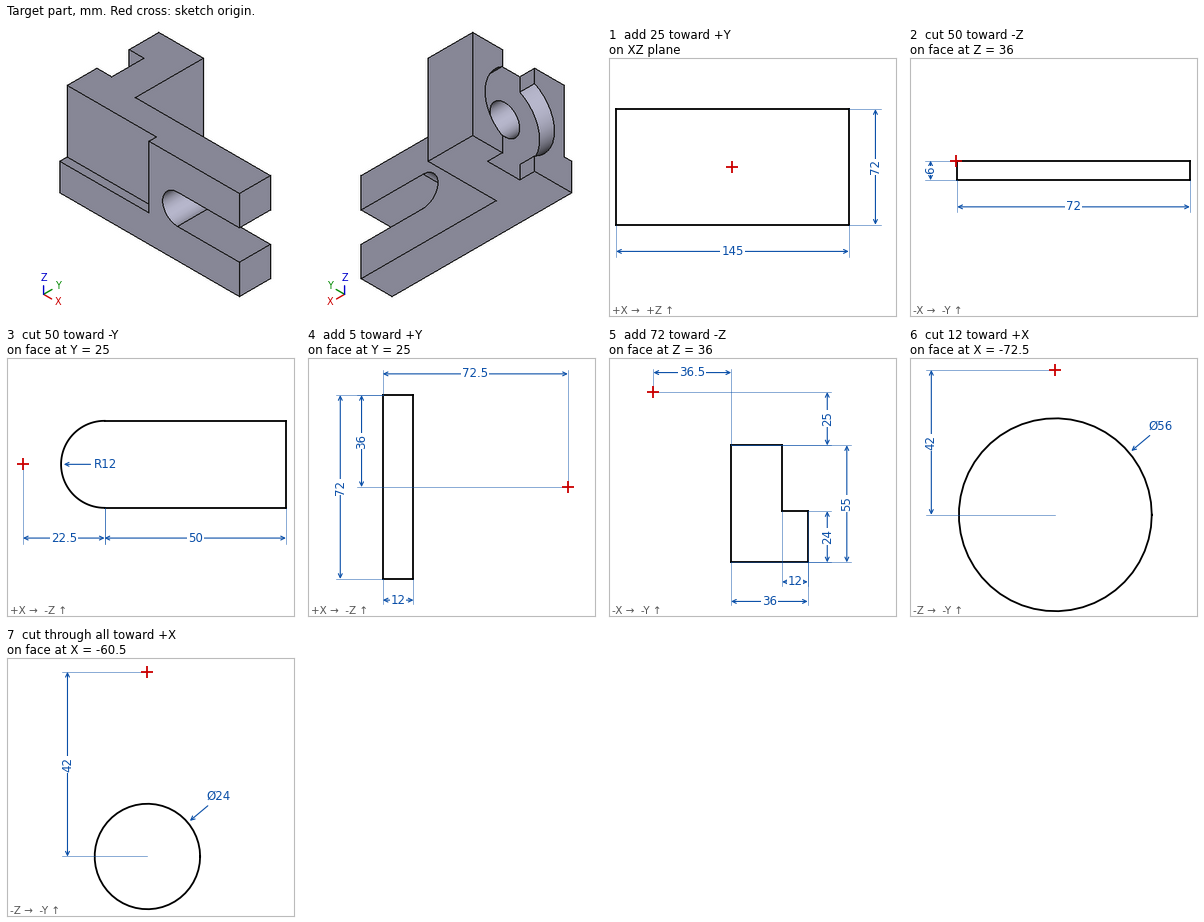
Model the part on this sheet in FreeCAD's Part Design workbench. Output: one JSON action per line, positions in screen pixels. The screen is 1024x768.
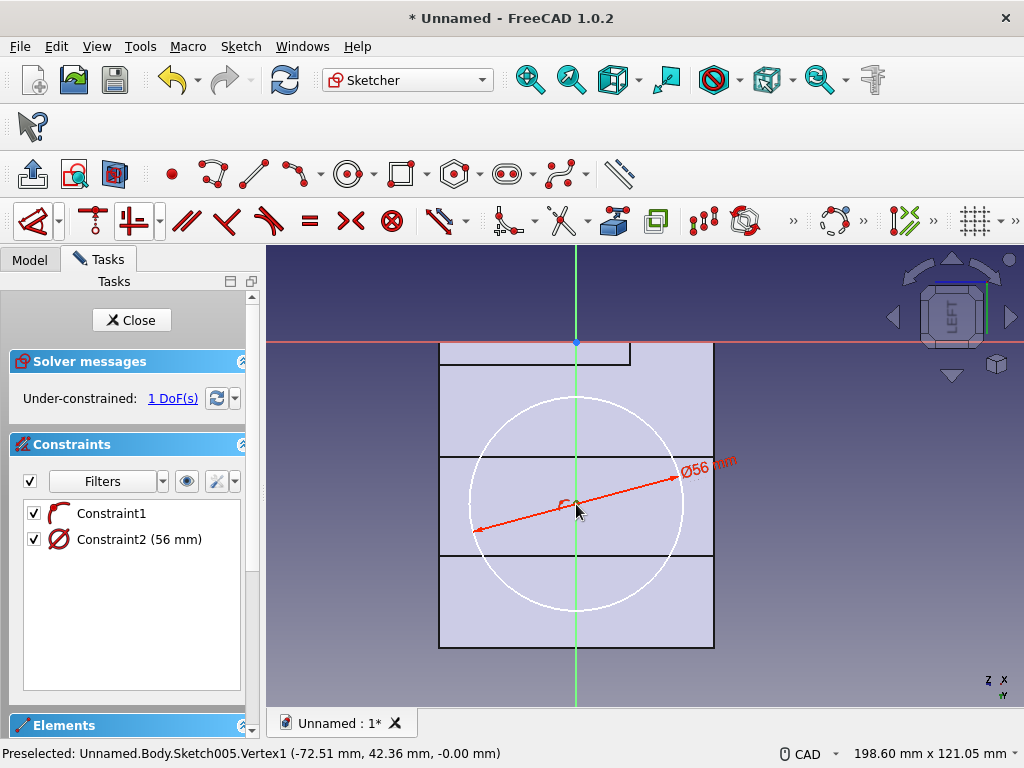
{"action": "key", "text": "i"}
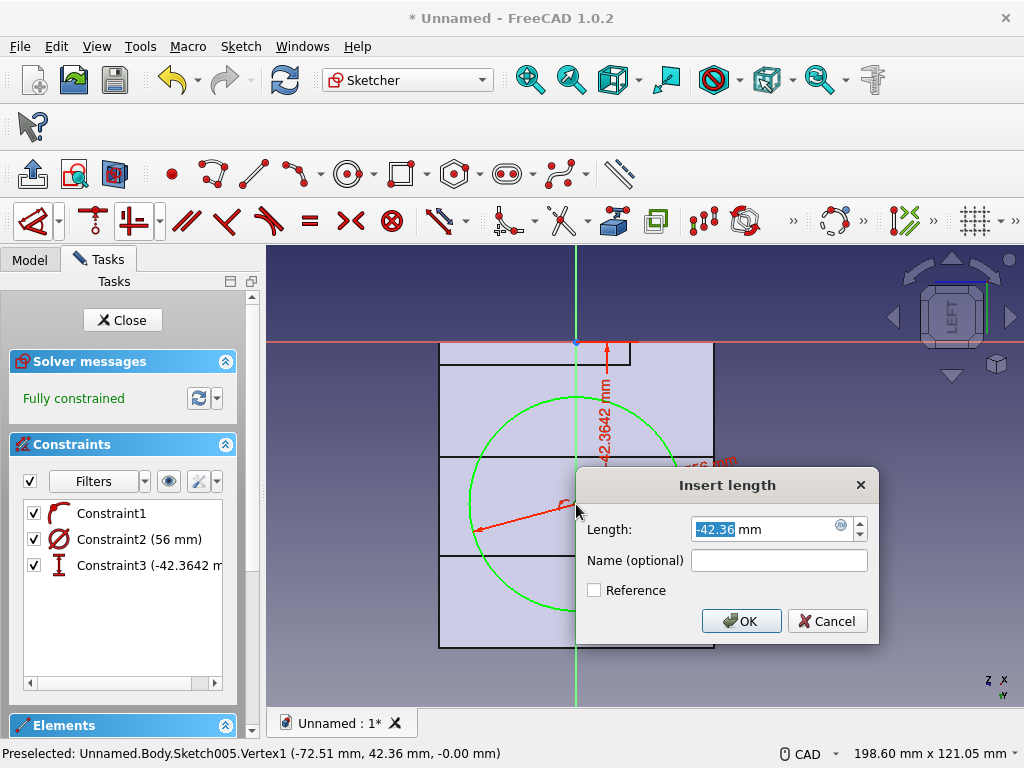
{"action": "type", "text": "-42"}
{"action": "key", "text": "Return"}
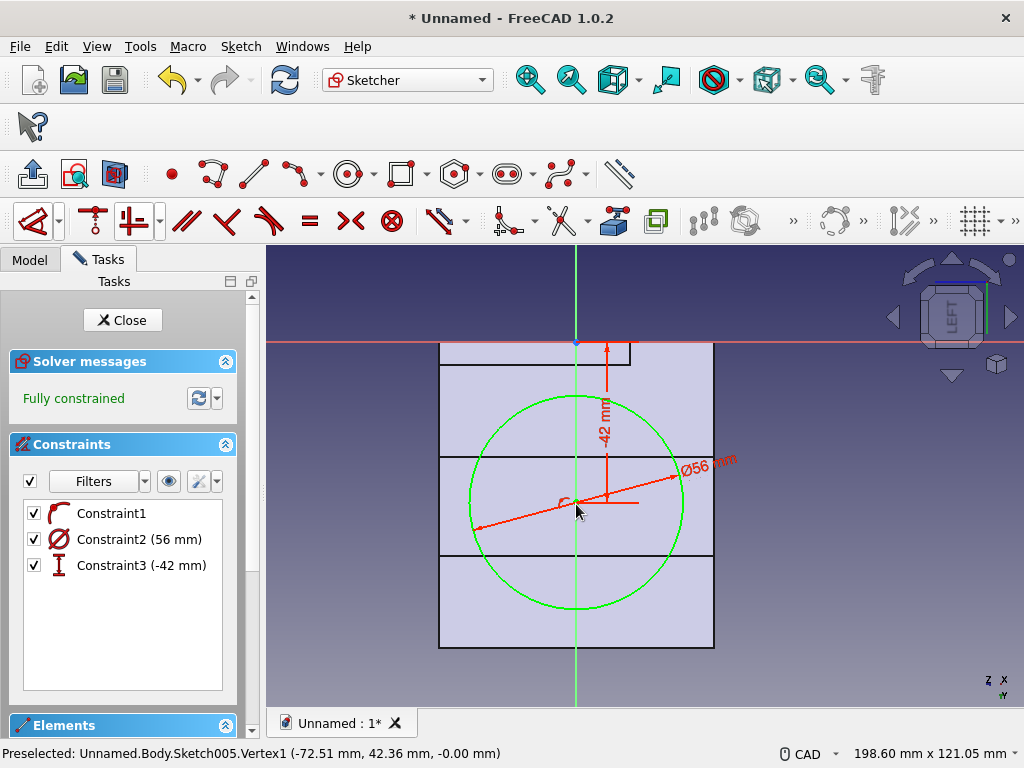
{"action": "left_click", "coordinate": [123, 320]}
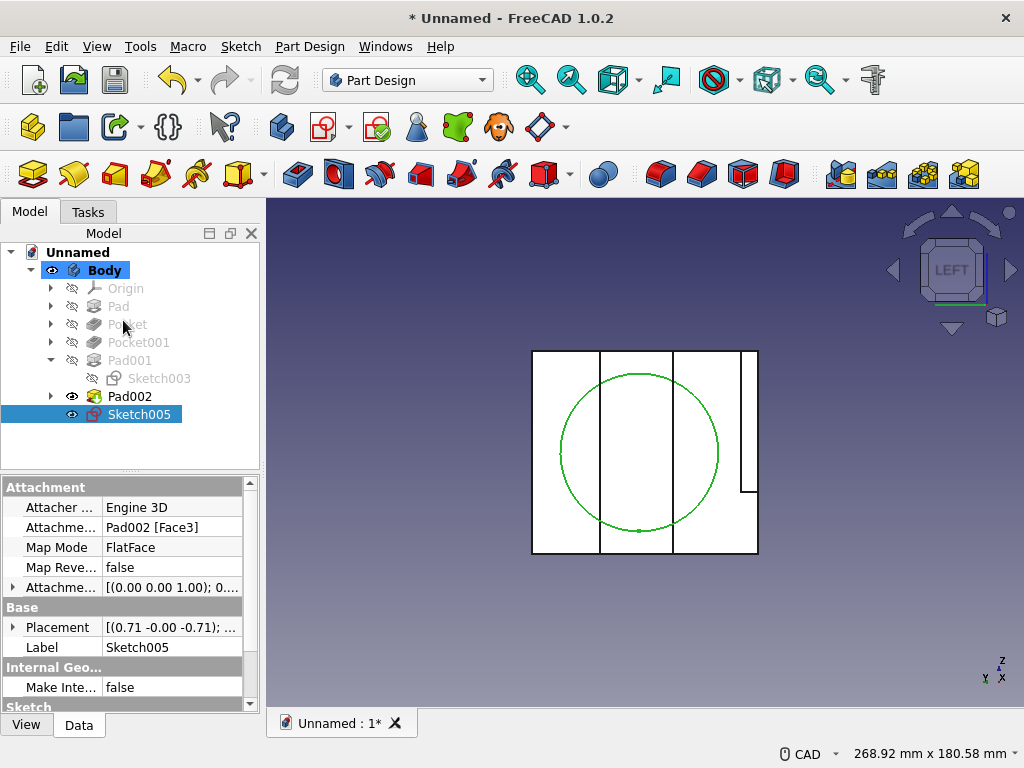
{"action": "left_click", "coordinate": [298, 174]}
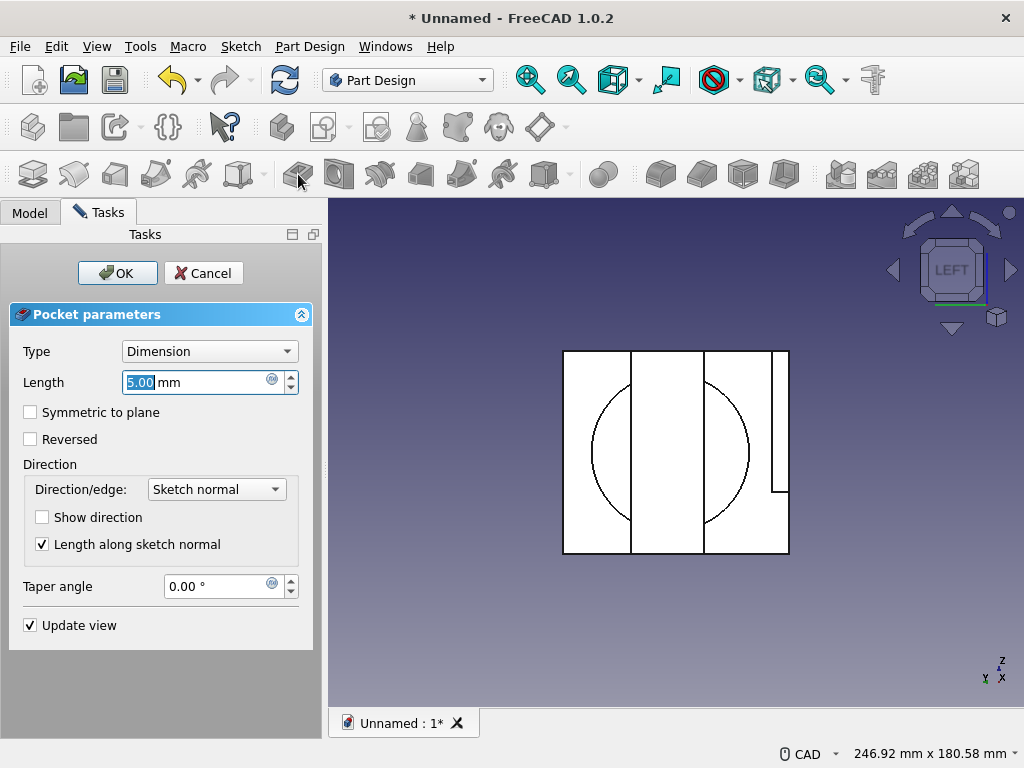
{"action": "type", "text": "12"}
{"action": "key", "text": "Tab"}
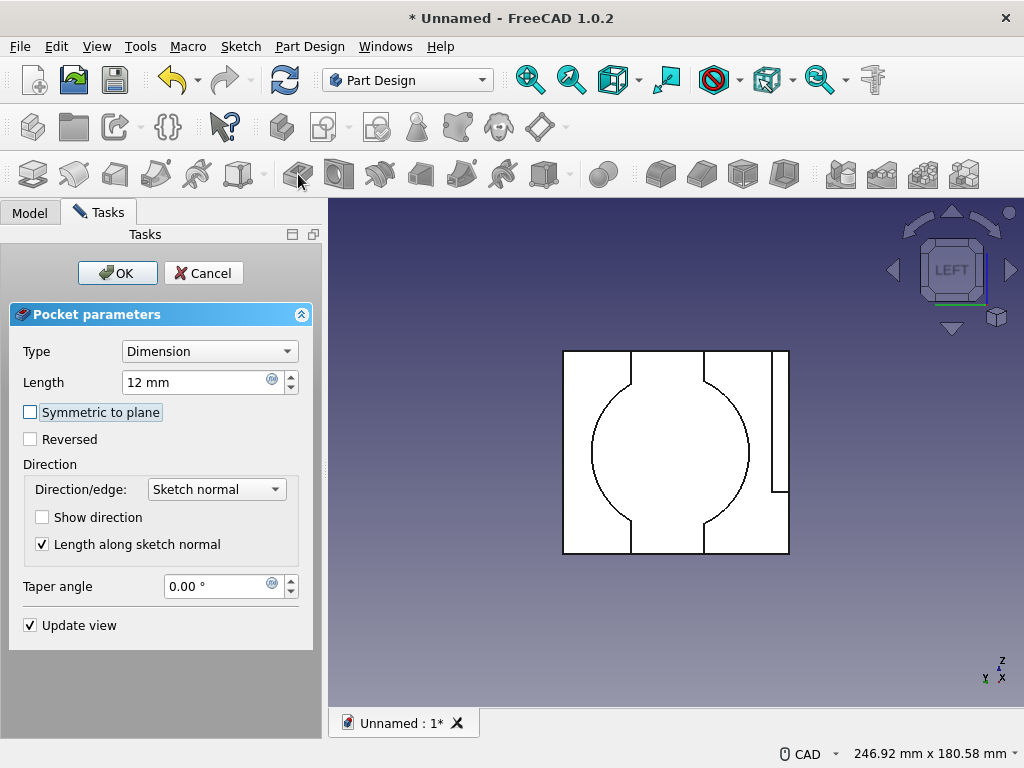
{"action": "left_click", "coordinate": [118, 273]}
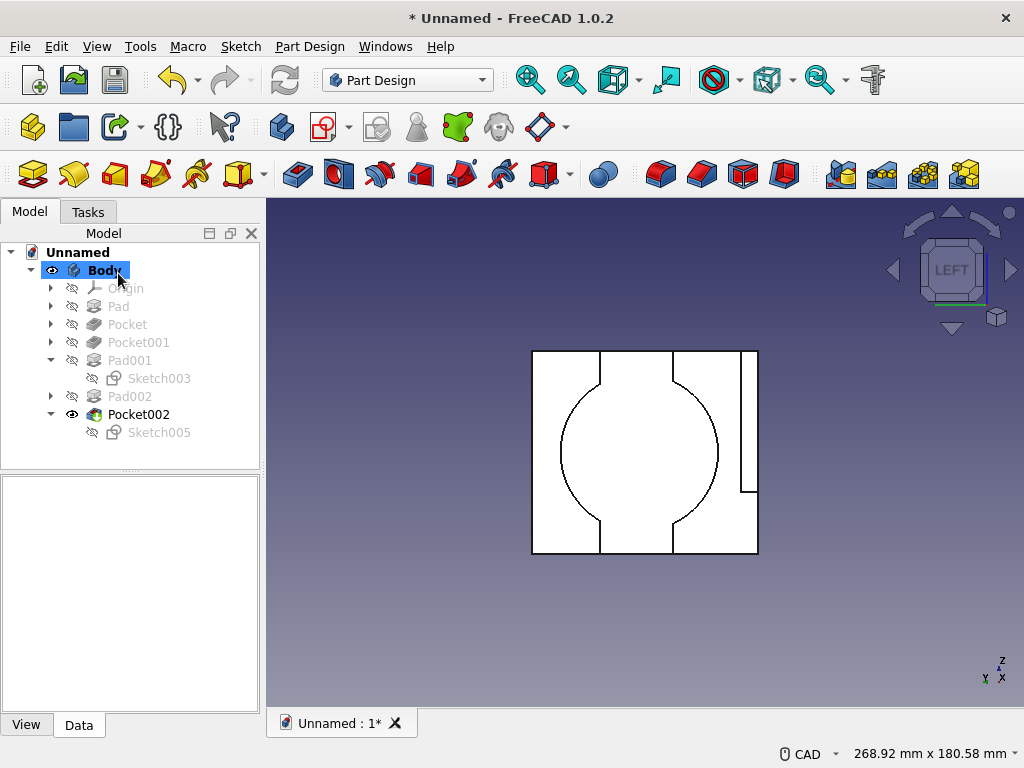
{"action": "left_click", "coordinate": [531, 80]}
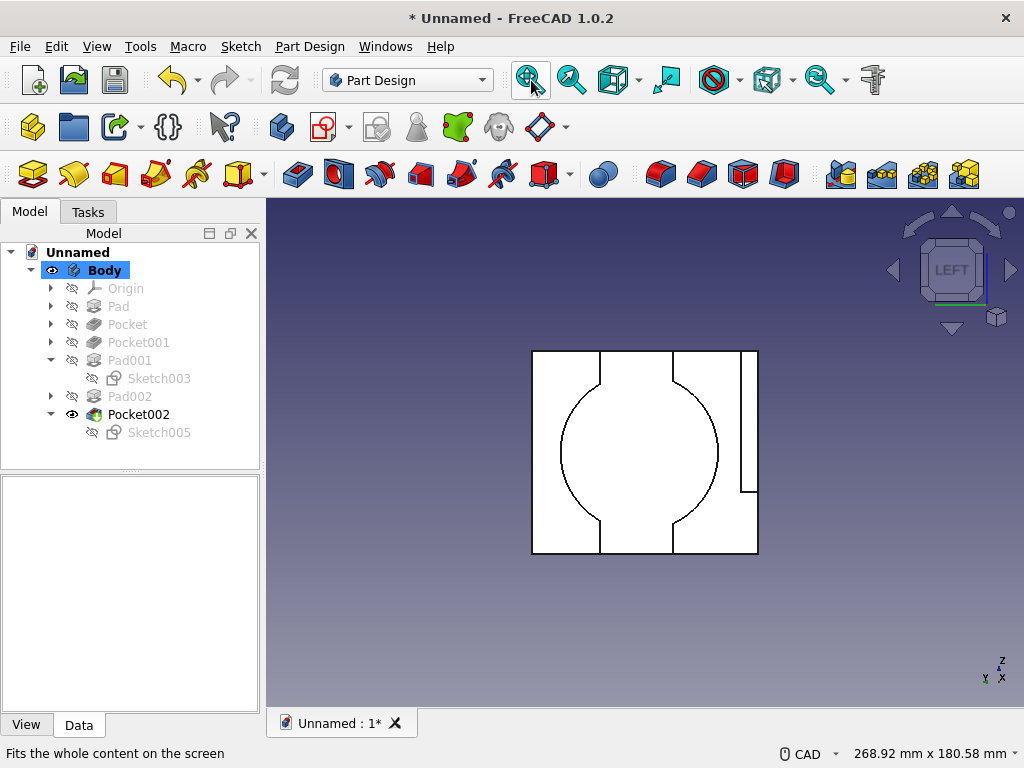
{"action": "left_click", "coordinate": [639, 451]}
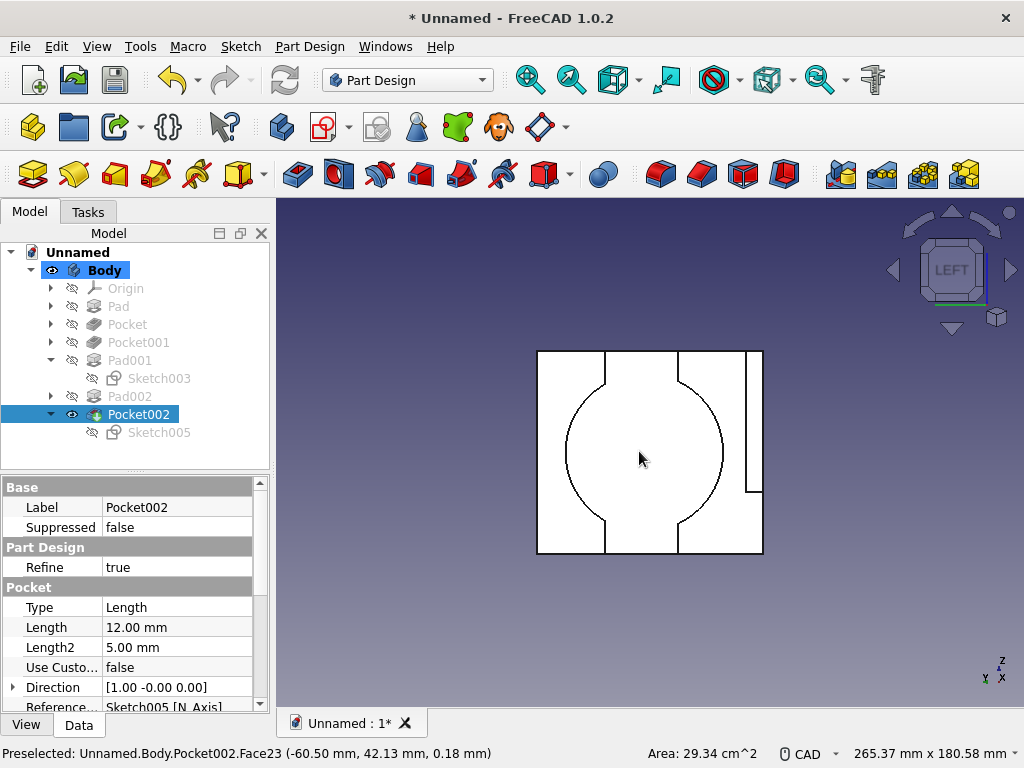
{"action": "left_click", "coordinate": [322, 128]}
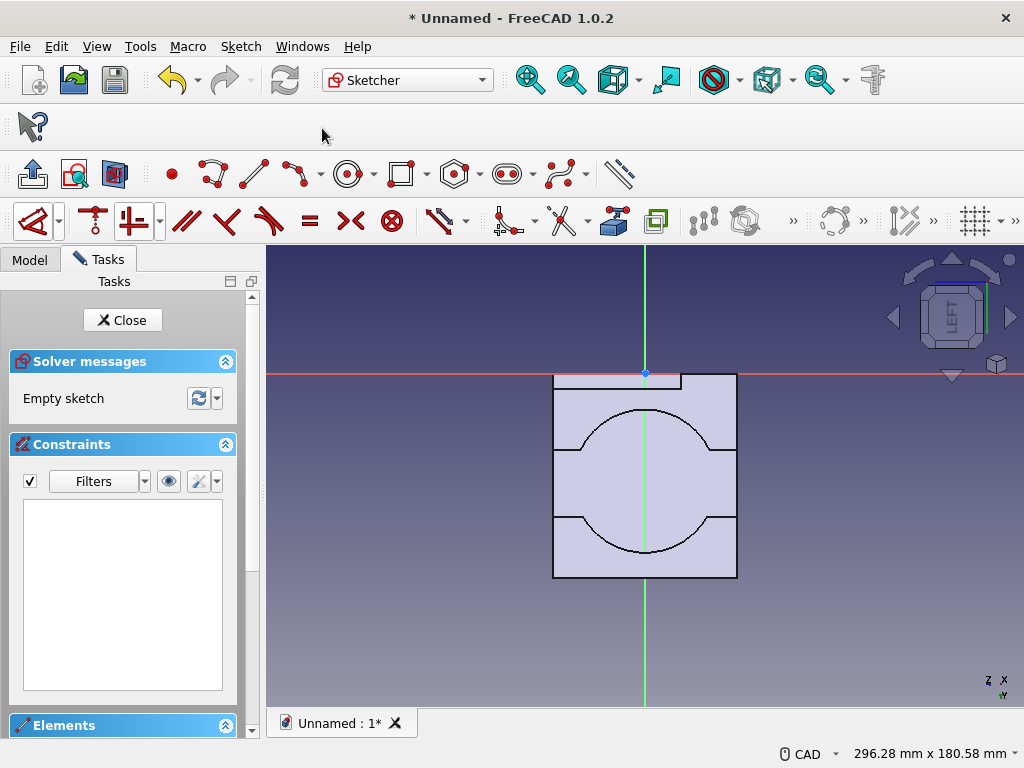
{"action": "scroll", "coordinate": [701, 416], "scroll_direction": "up", "scroll_amount": 4}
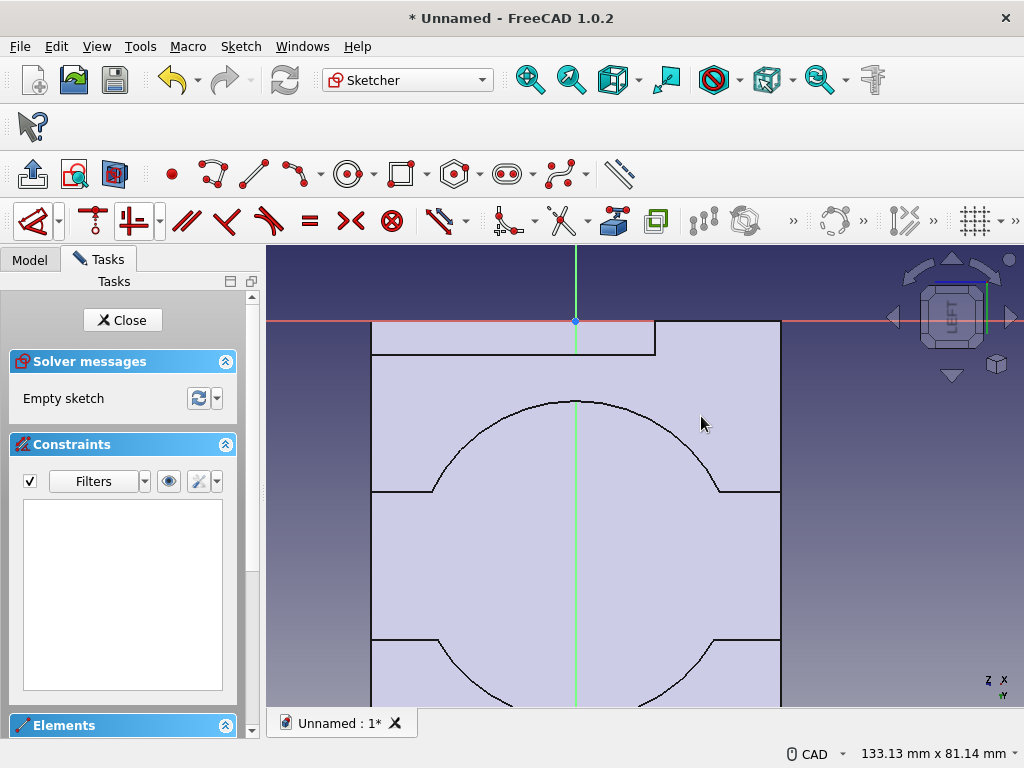
{"action": "left_click", "coordinate": [348, 174]}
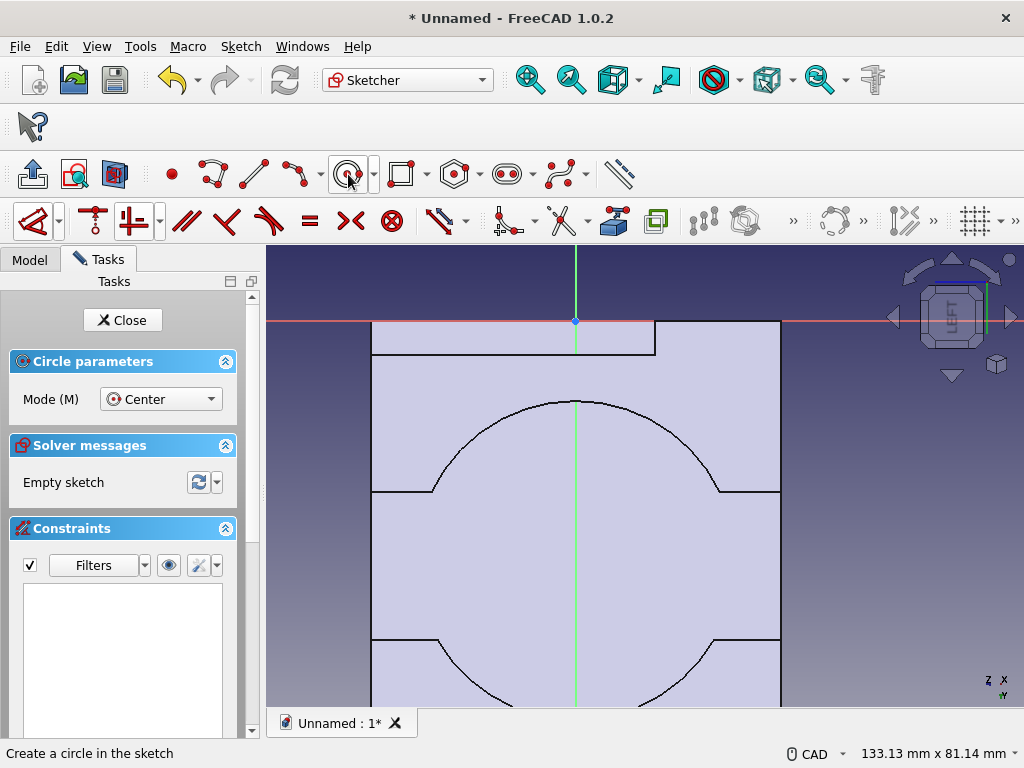
{"action": "left_click", "coordinate": [576, 560]}
{"action": "left_click", "coordinate": [624, 512]}
{"action": "key", "text": "Escape"}